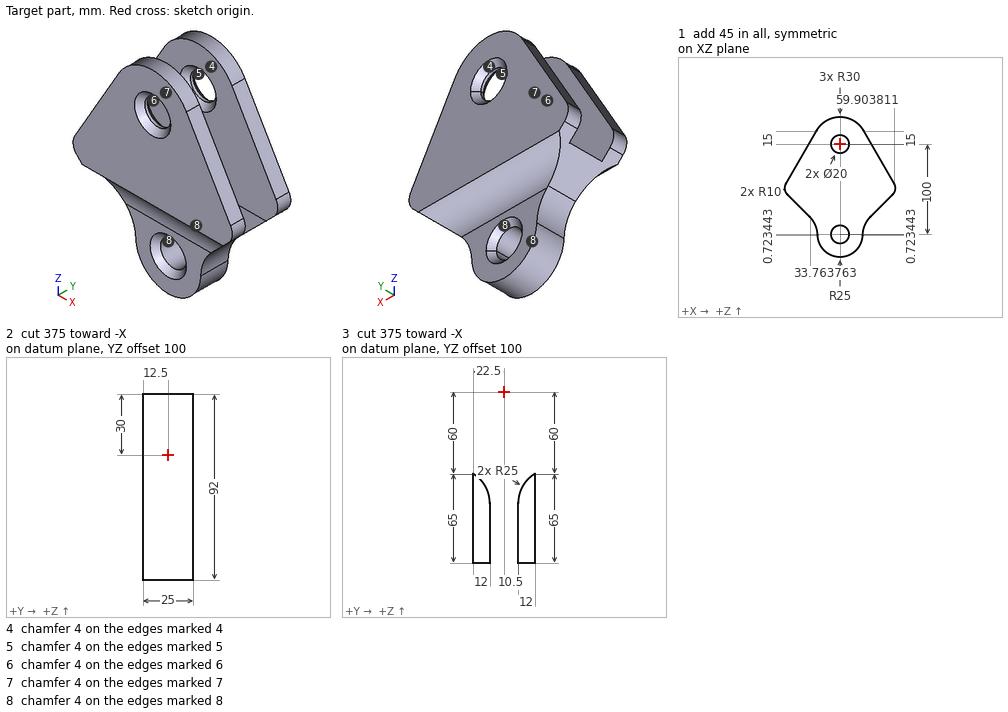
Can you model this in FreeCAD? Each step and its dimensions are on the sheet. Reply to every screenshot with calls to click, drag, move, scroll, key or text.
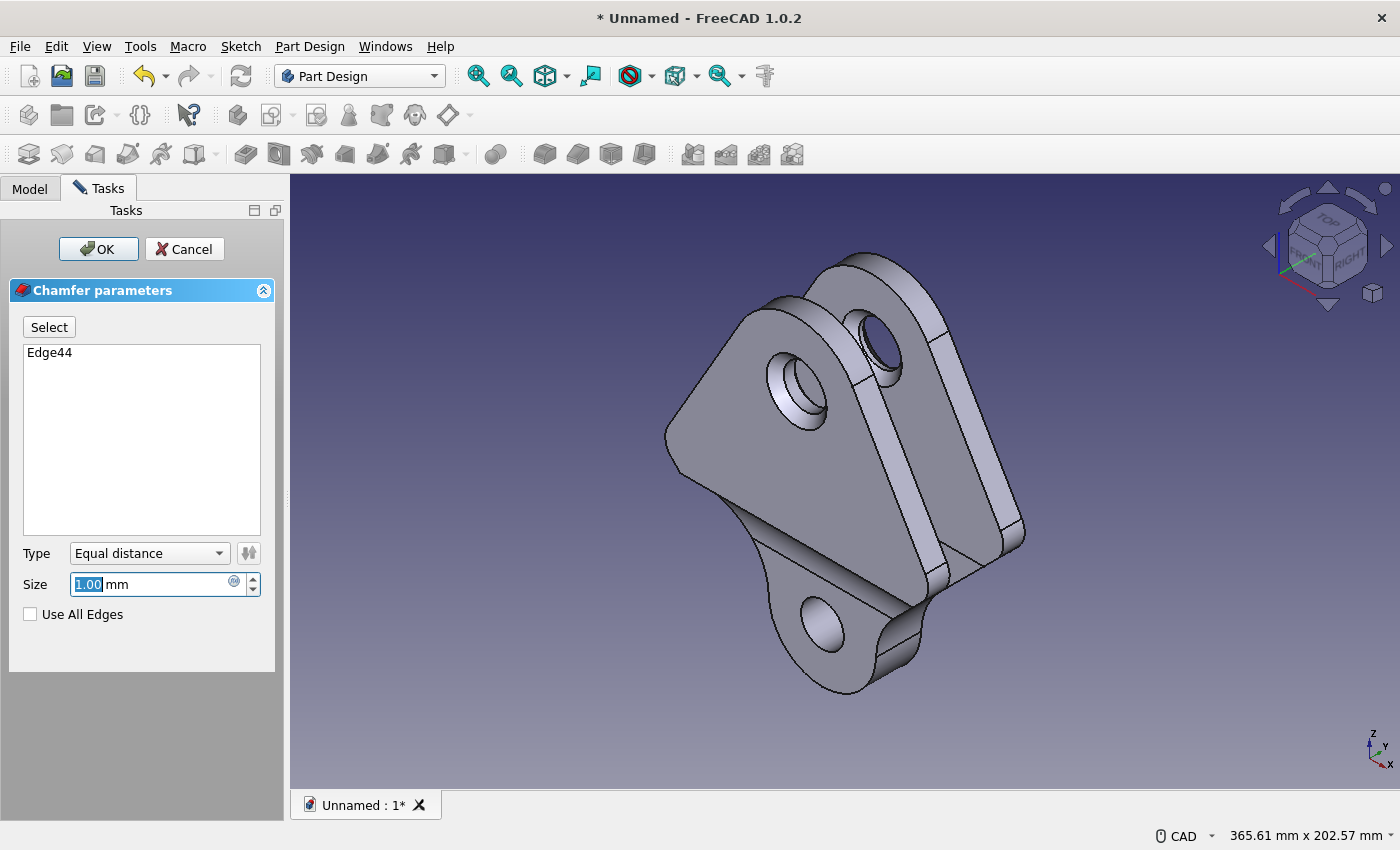
text(4)
key(Tab)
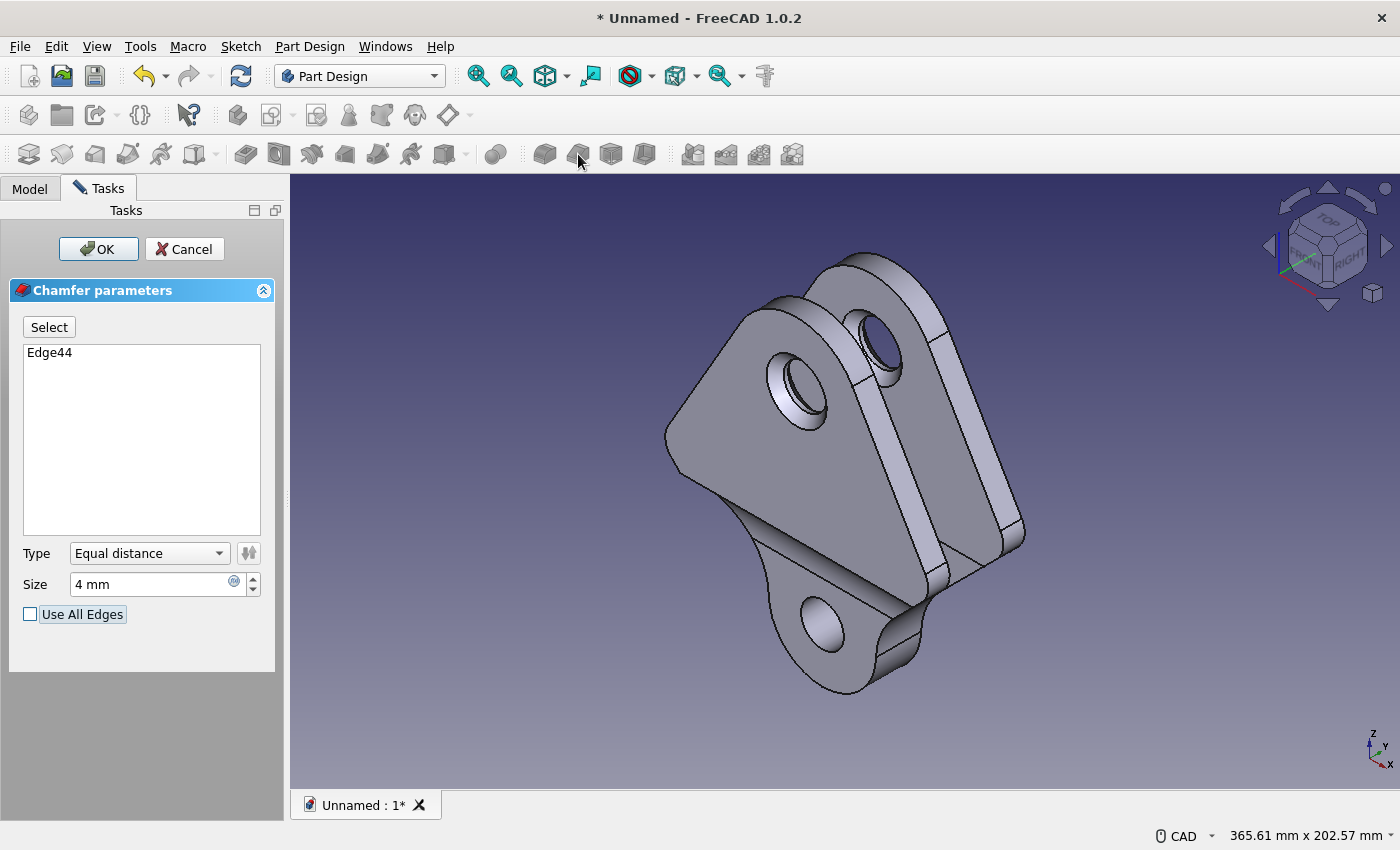
click(99, 249)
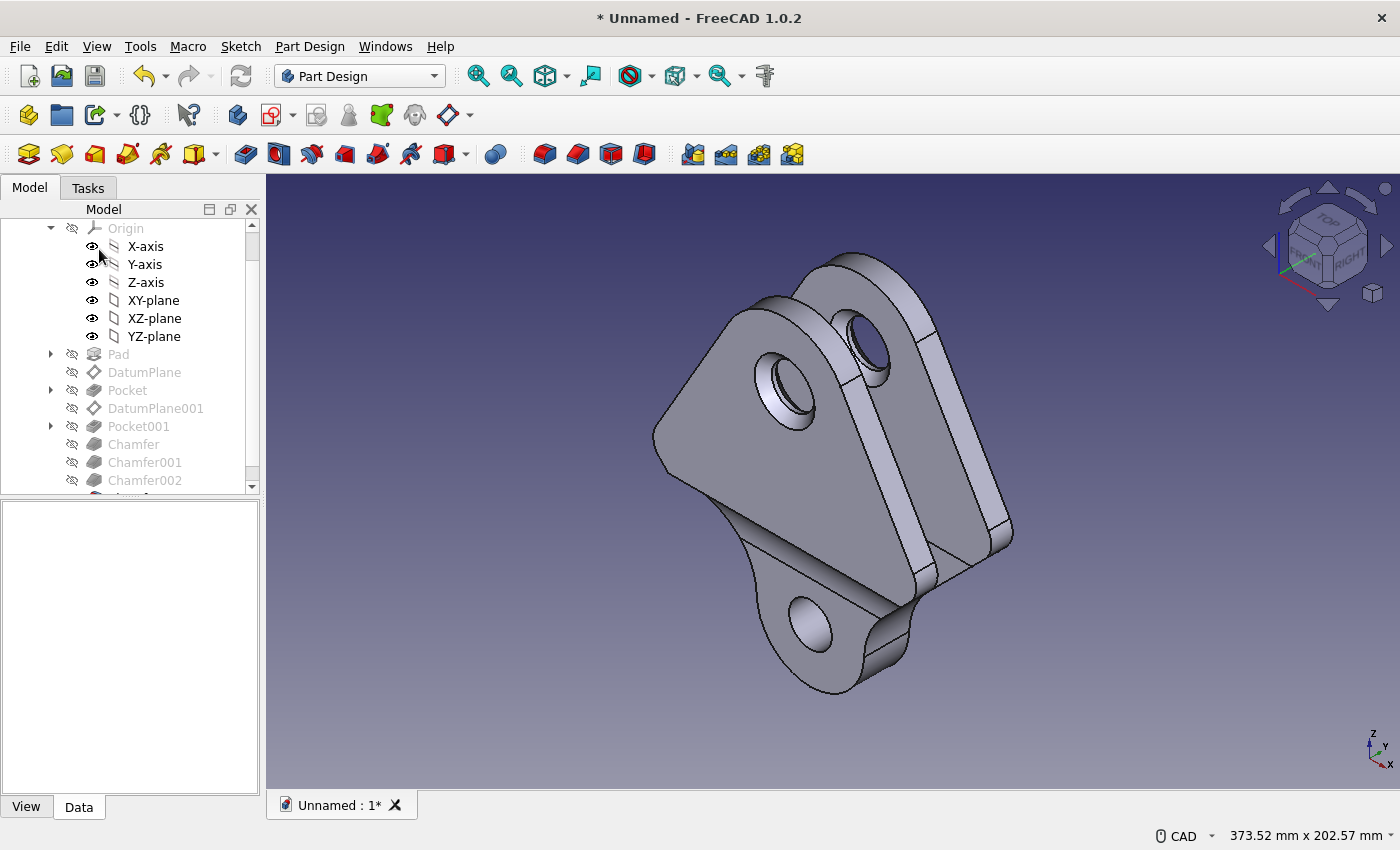
click(789, 611)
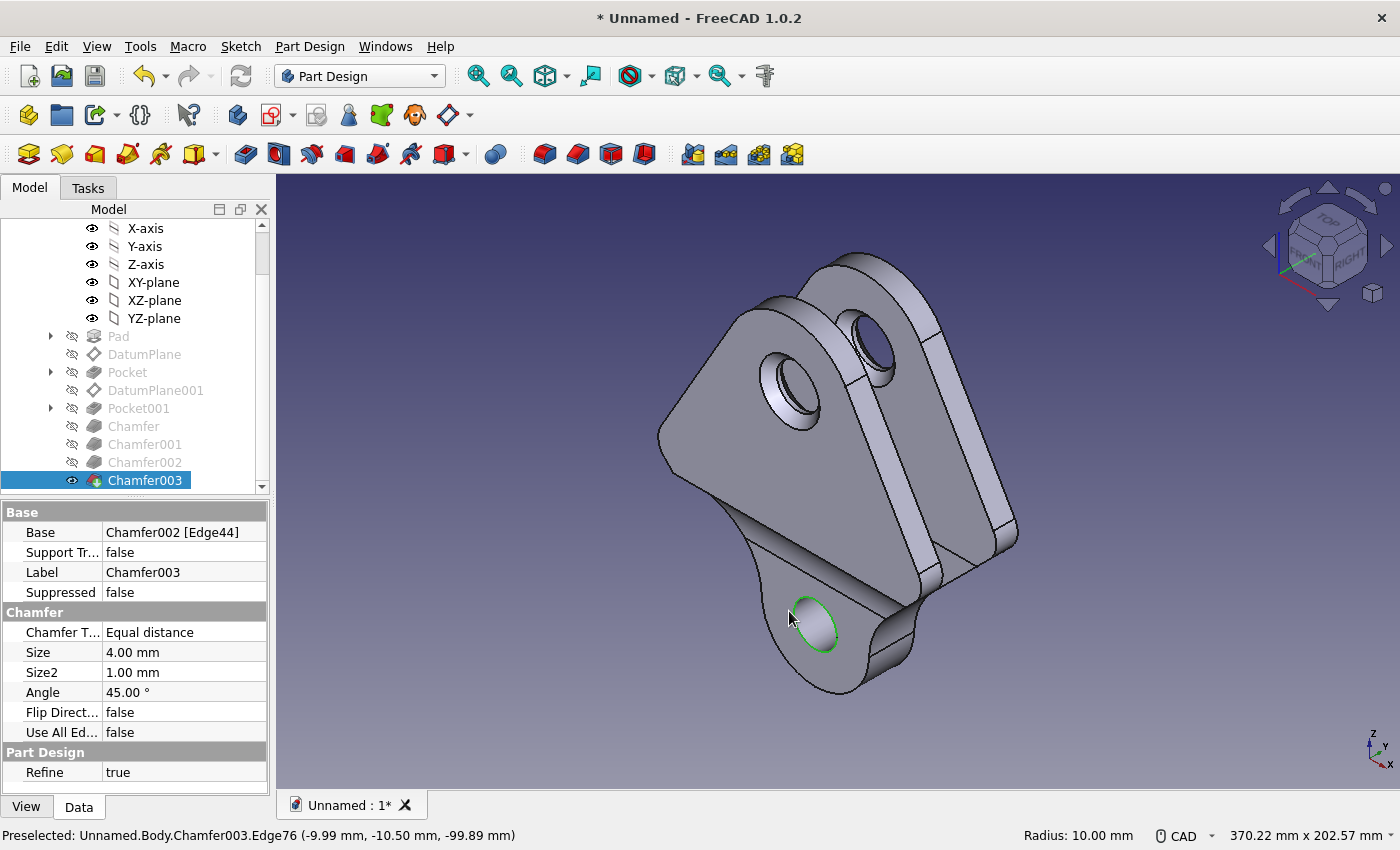
key(2)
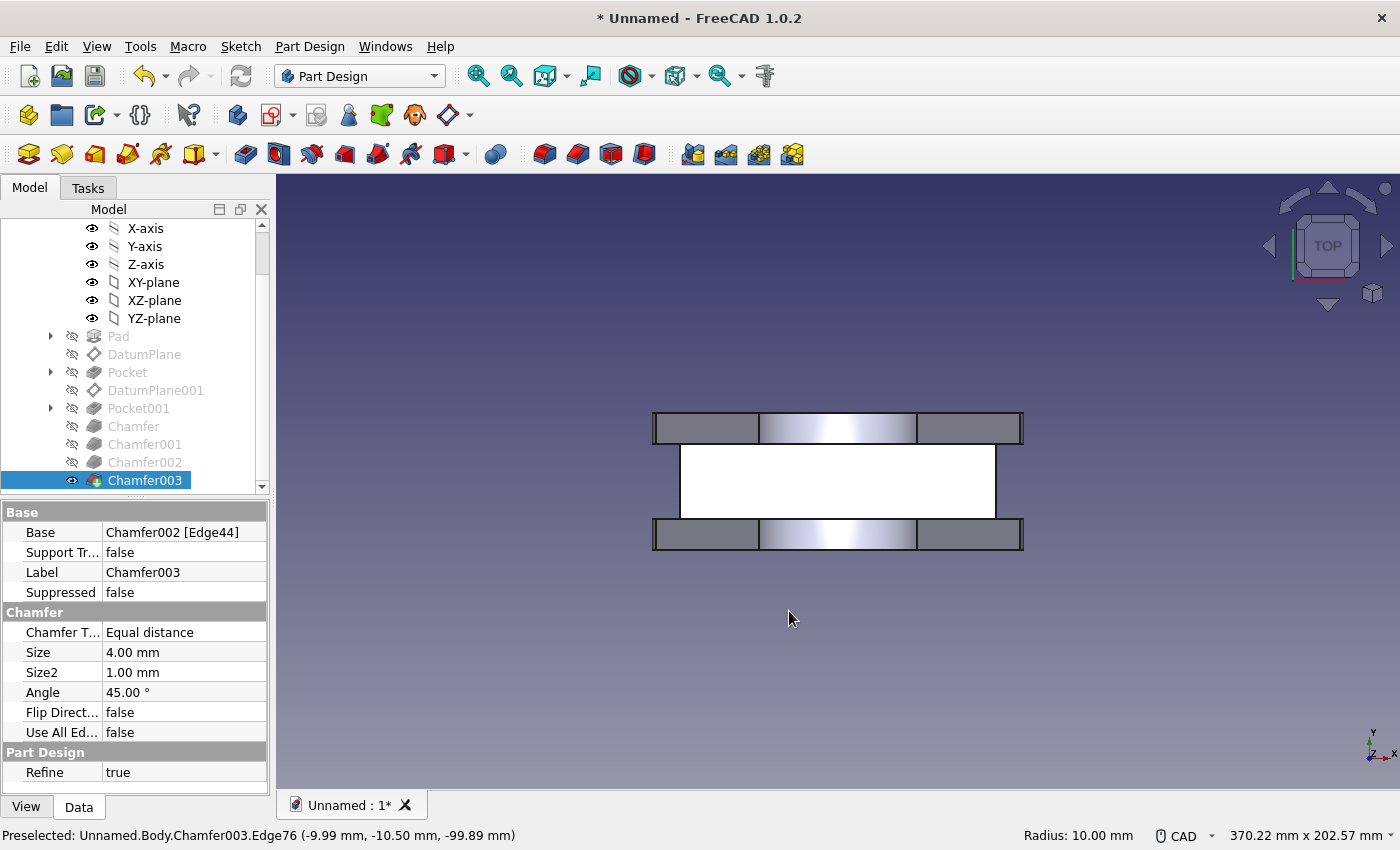
click(479, 76)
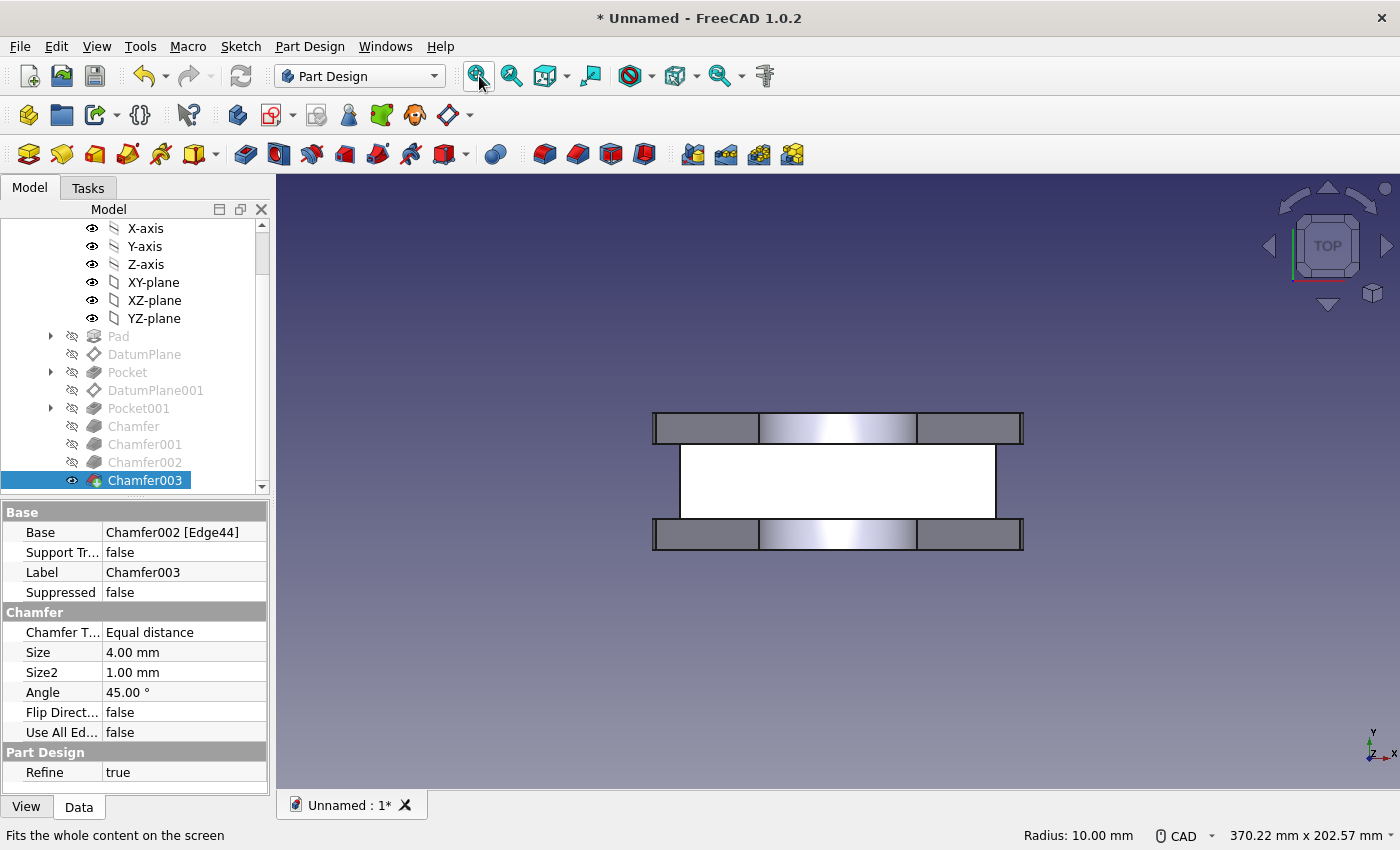
key(0)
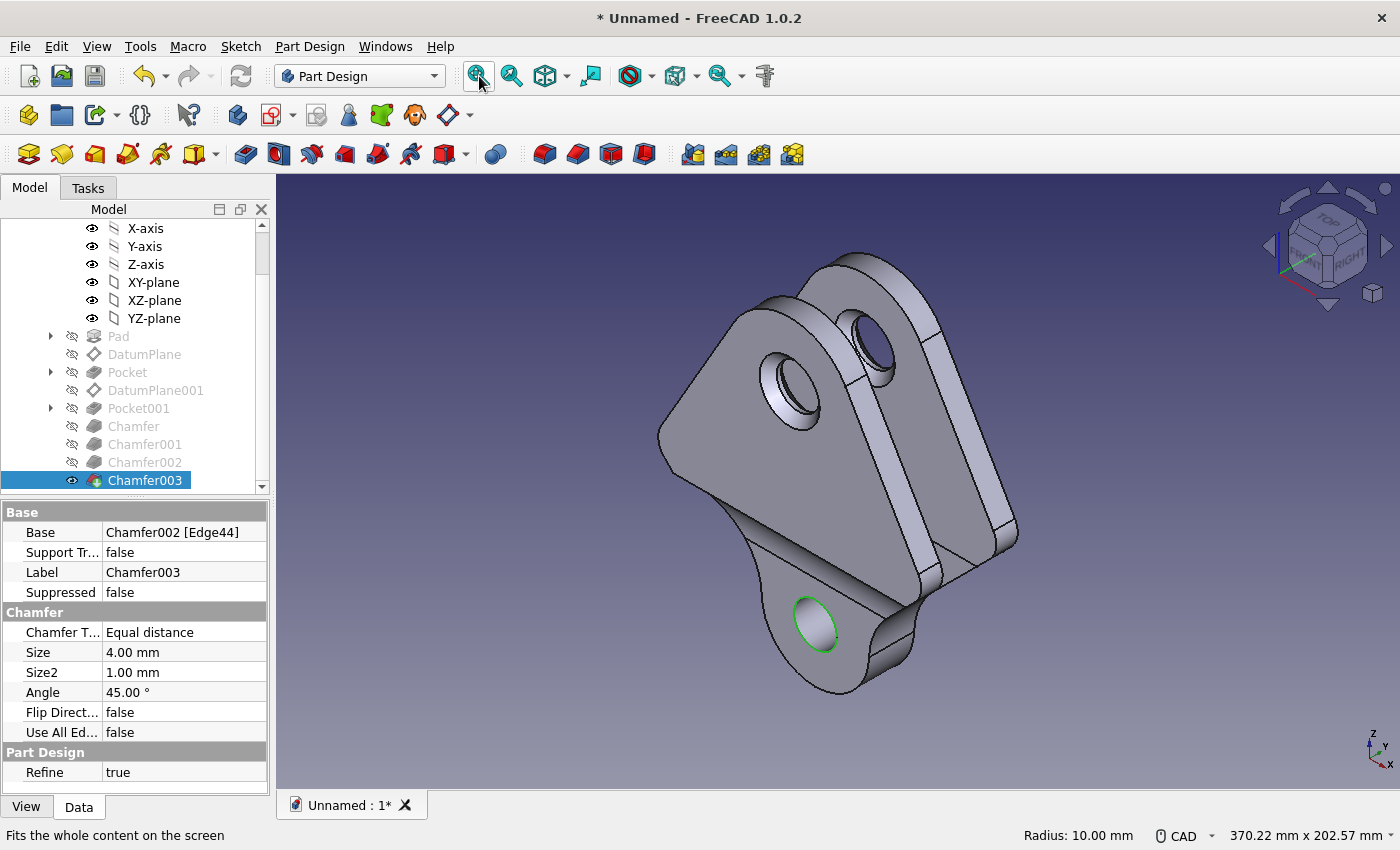
key(1)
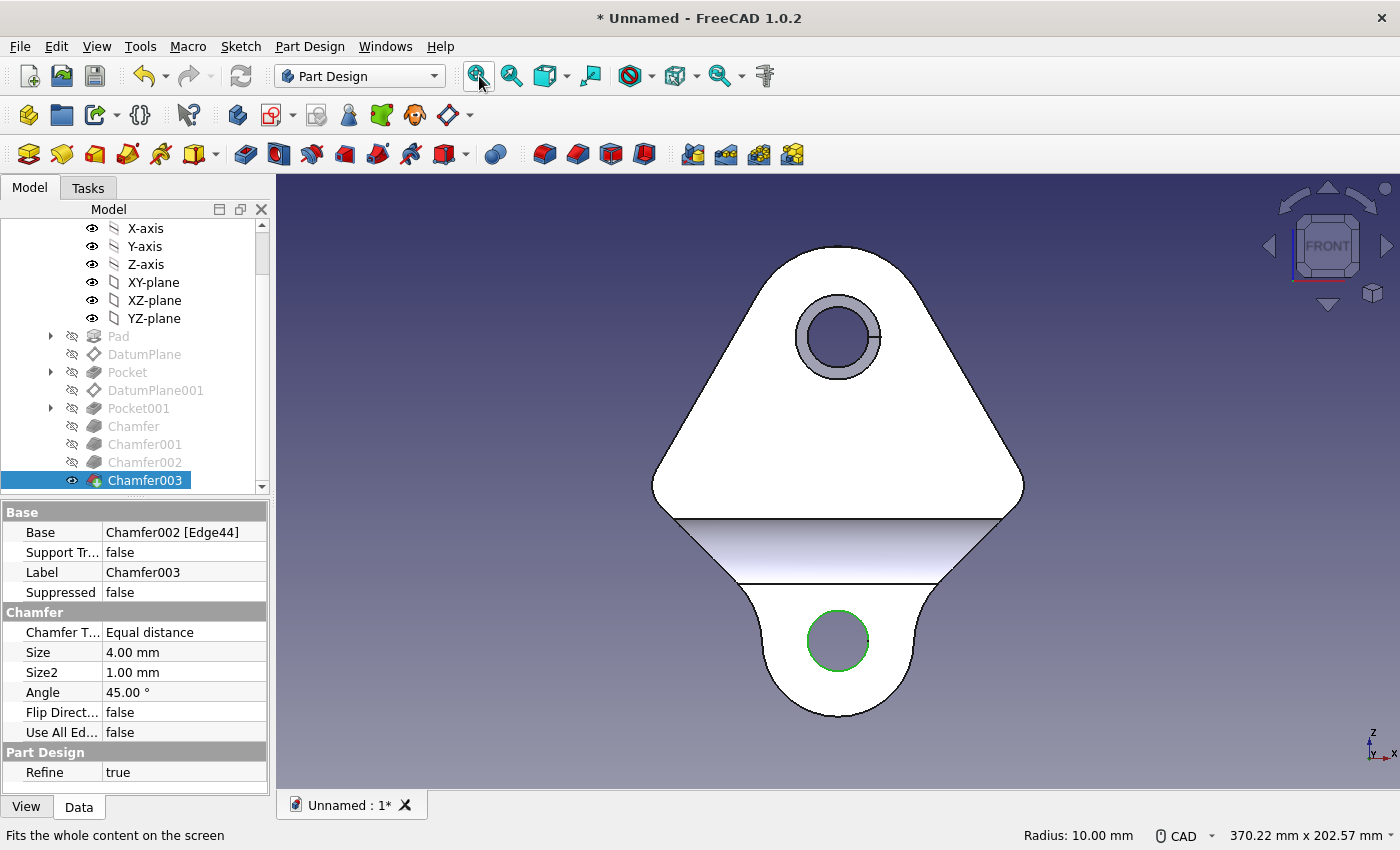
key(3)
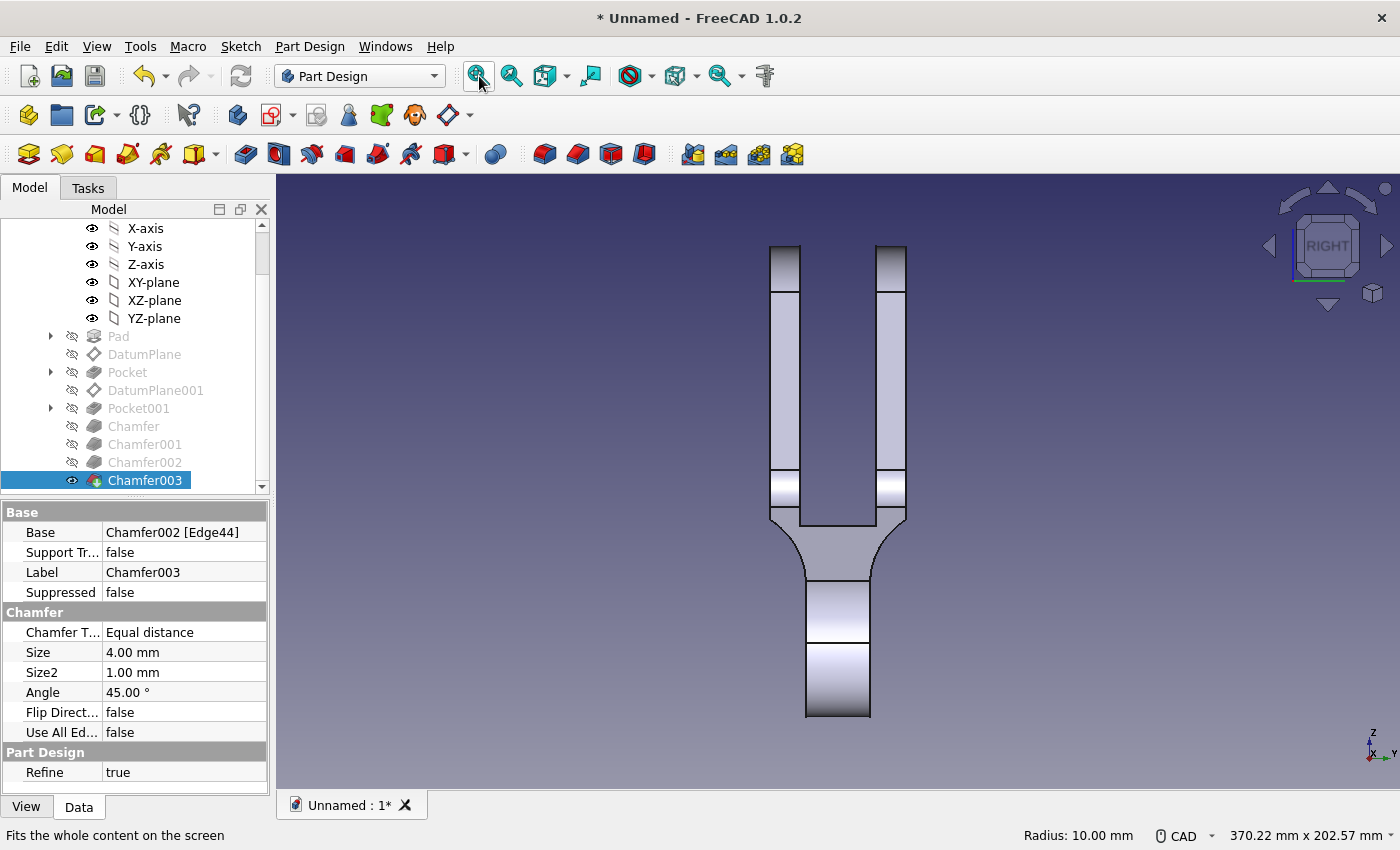
key(5)